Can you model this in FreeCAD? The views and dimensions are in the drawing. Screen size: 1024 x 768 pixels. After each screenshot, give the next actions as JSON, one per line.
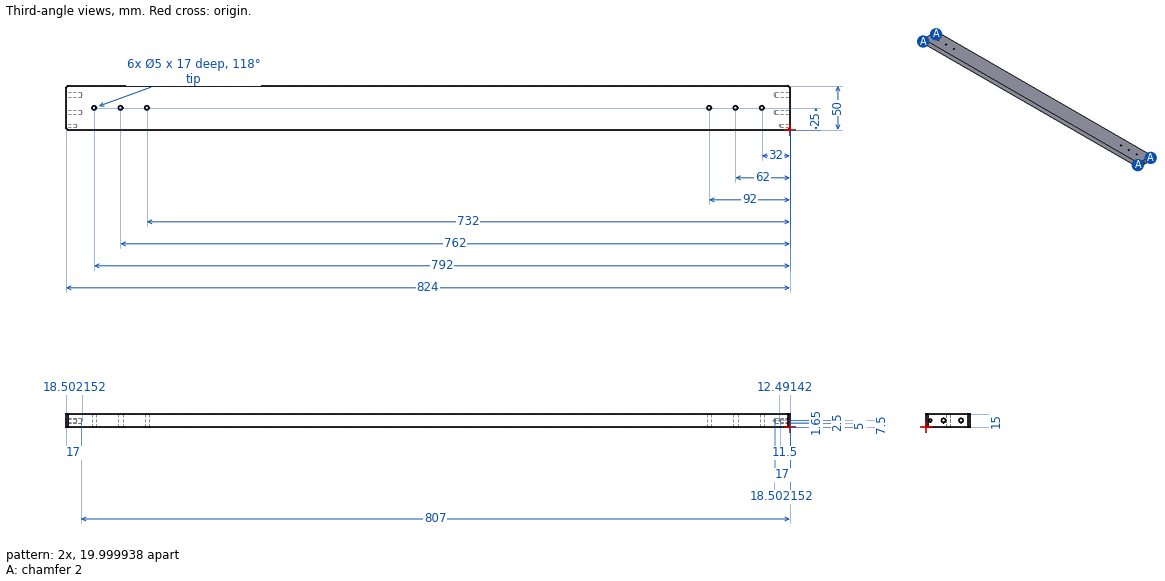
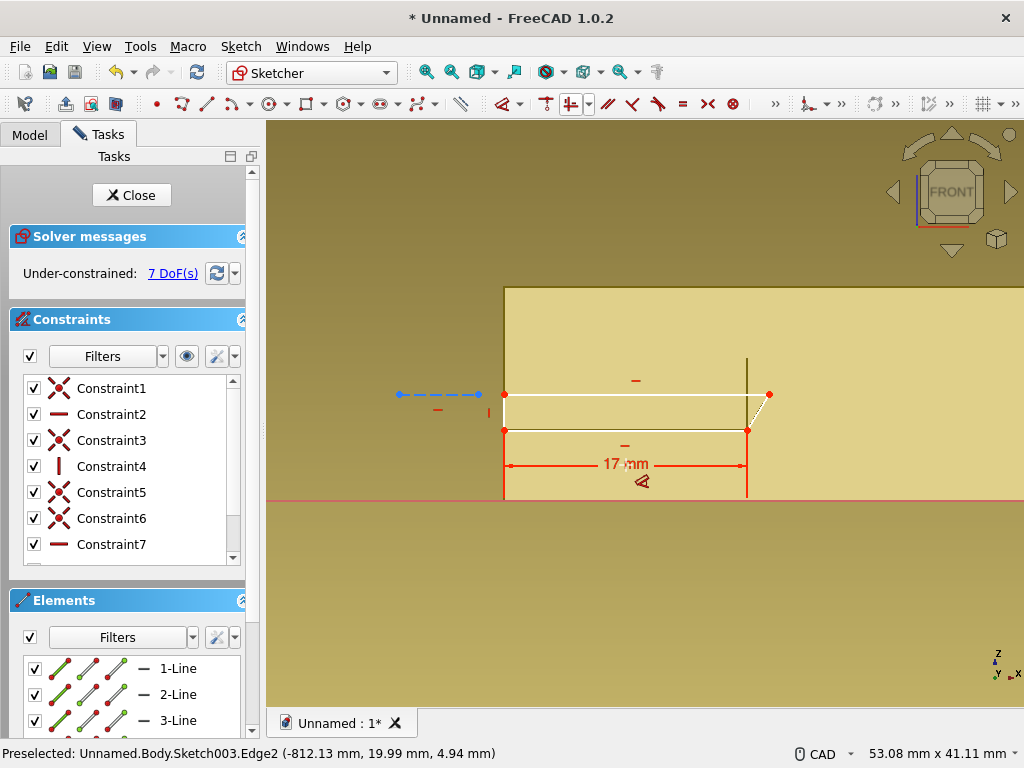
{"action": "left_click", "coordinate": [747, 431]}
{"action": "left_click", "coordinate": [713, 466]}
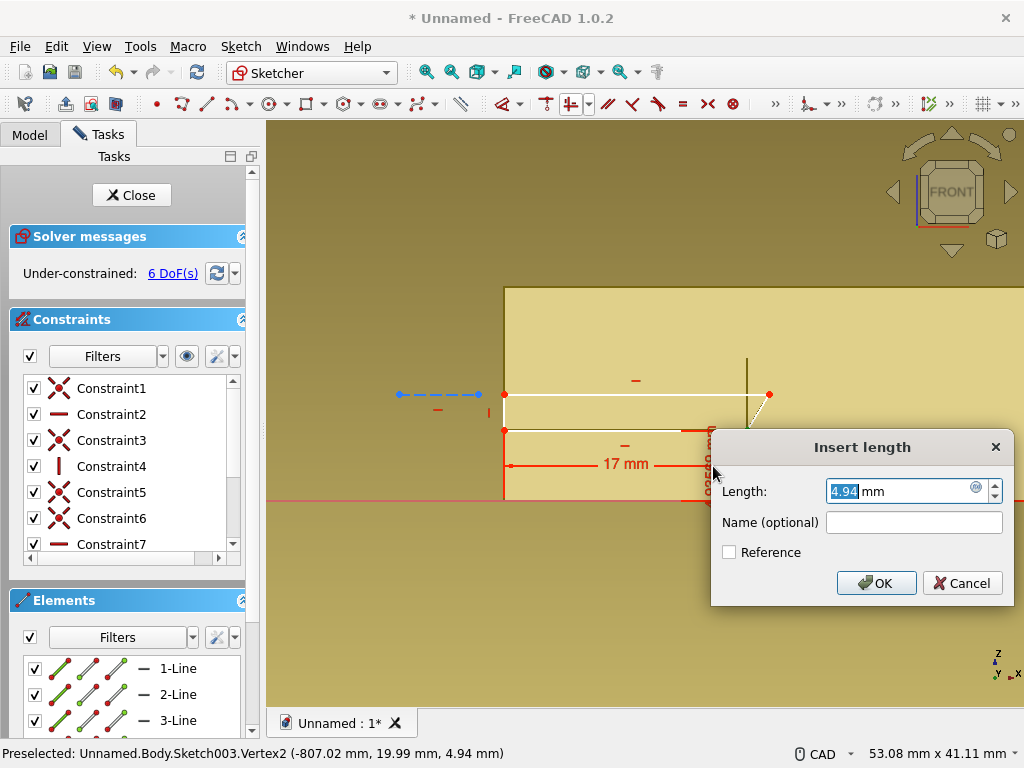
{"action": "type", "text": "5"}
{"action": "key", "text": "Return"}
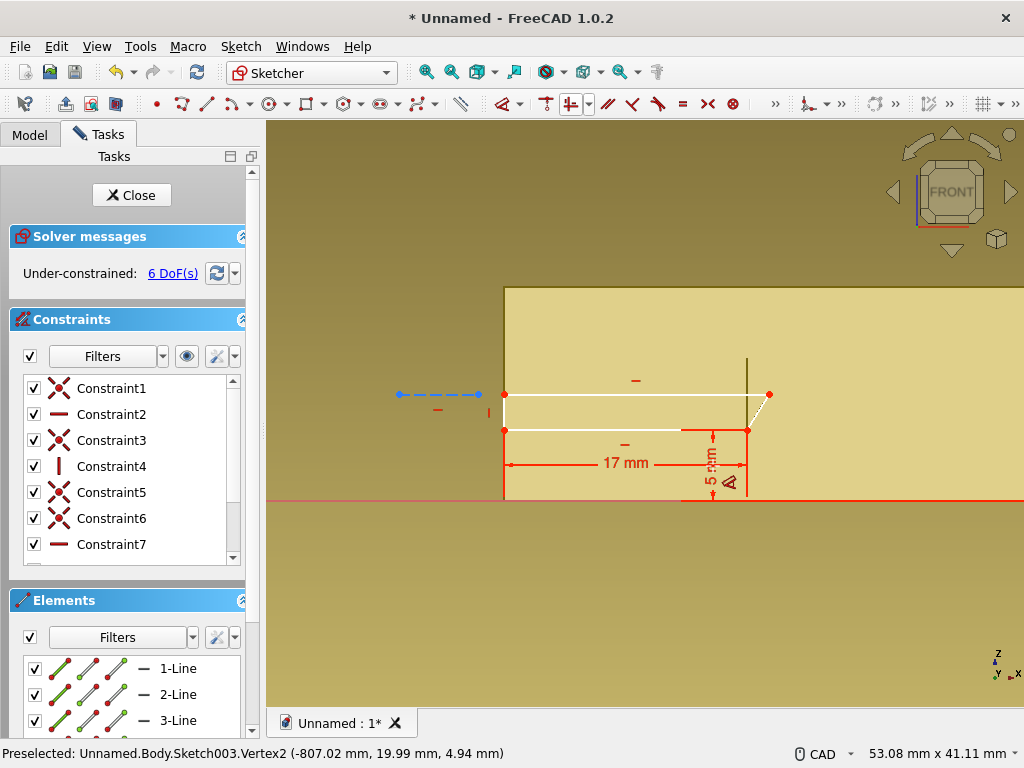
{"action": "scroll", "coordinate": [504, 420], "scroll_direction": "up", "scroll_amount": 2}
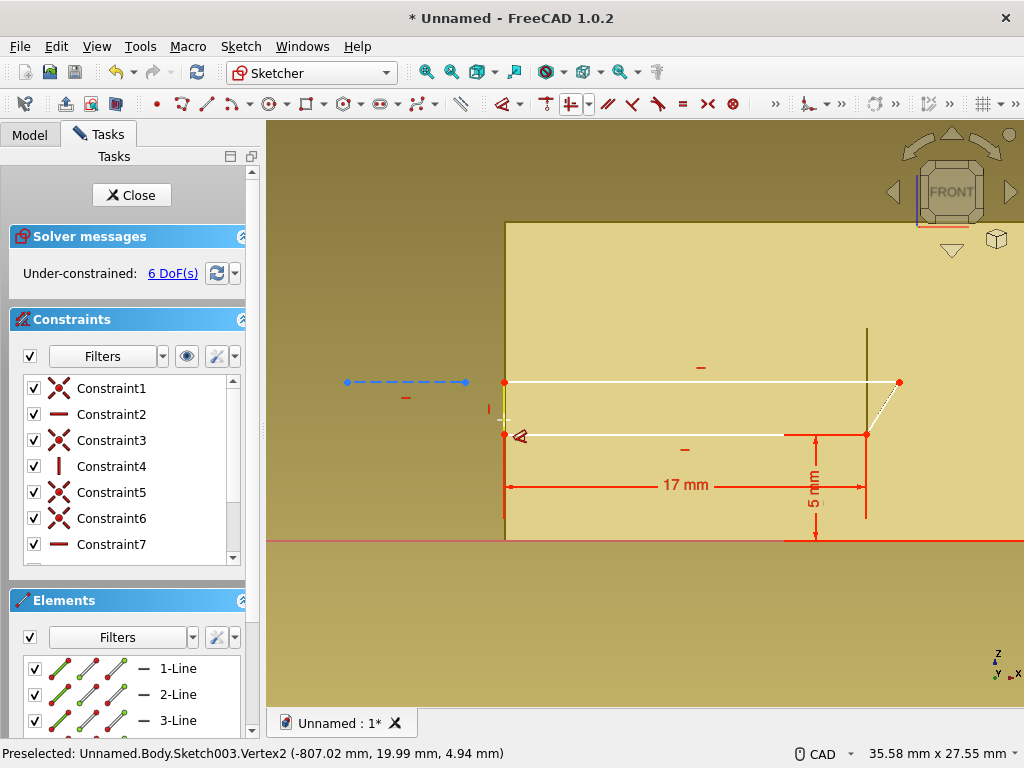
{"action": "left_click", "coordinate": [504, 419]}
{"action": "left_click", "coordinate": [470, 409]}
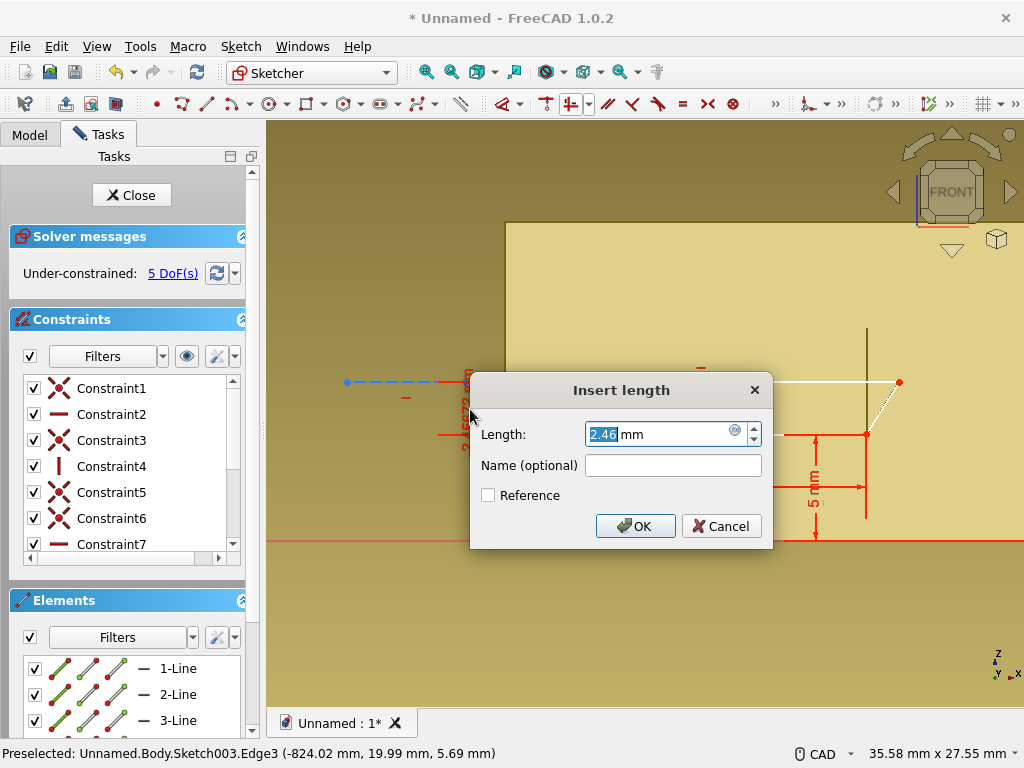
{"action": "type", "text": "2.5"}
{"action": "key", "text": "Return"}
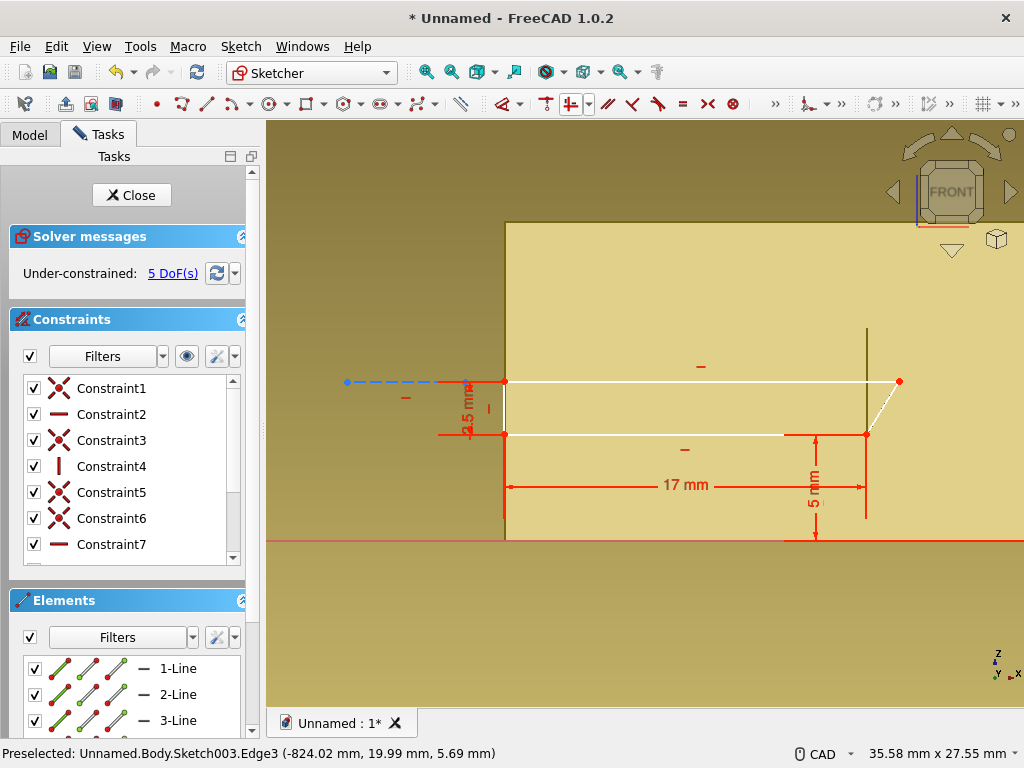
{"action": "scroll", "coordinate": [482, 424], "scroll_direction": "down", "scroll_amount": 2}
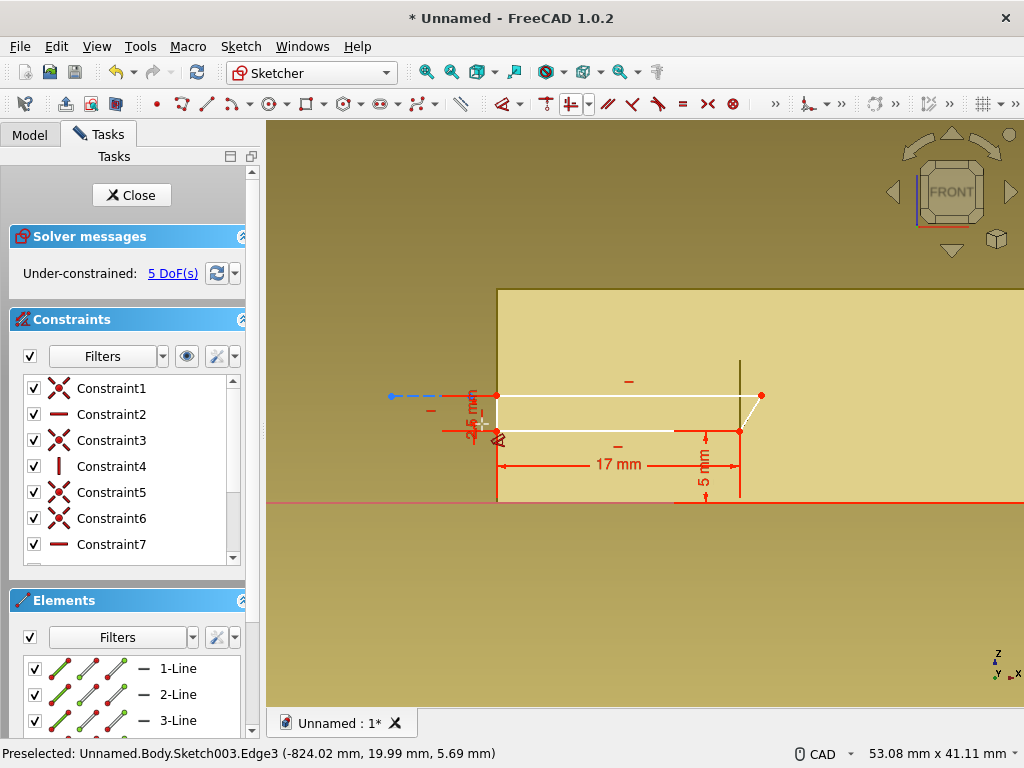
{"action": "left_click", "coordinate": [740, 431]}
{"action": "left_click", "coordinate": [799, 537]}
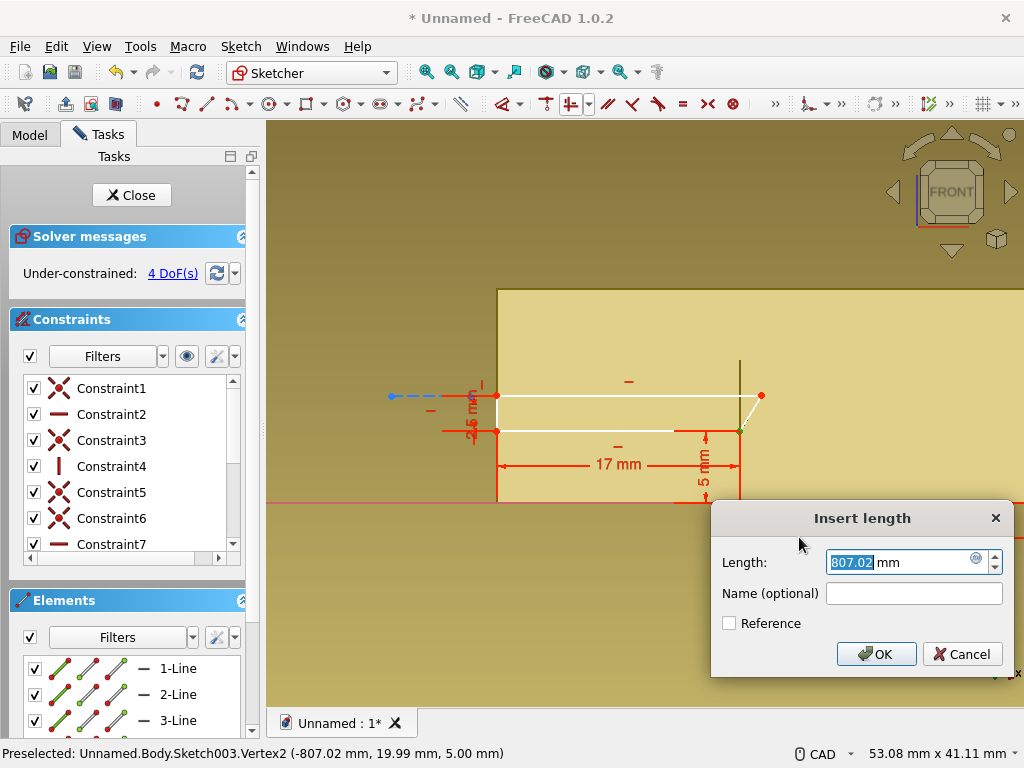
{"action": "type", "text": "807"}
{"action": "key", "text": "Return"}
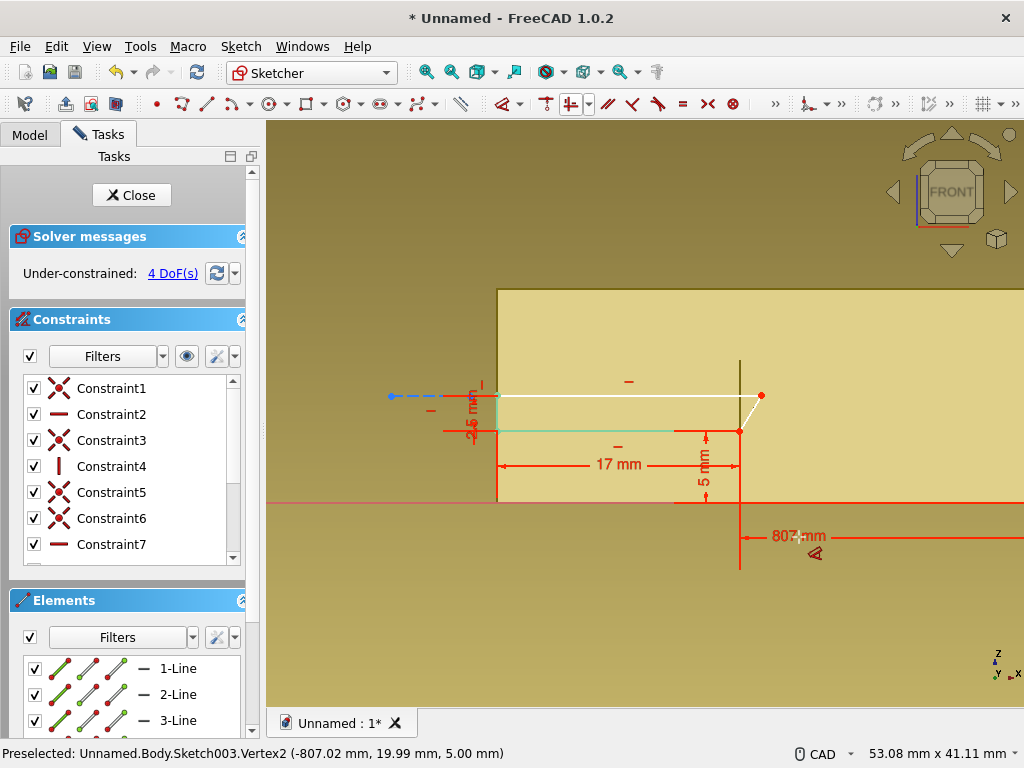
{"action": "left_click", "coordinate": [471, 396]}
{"action": "left_click", "coordinate": [437, 450]}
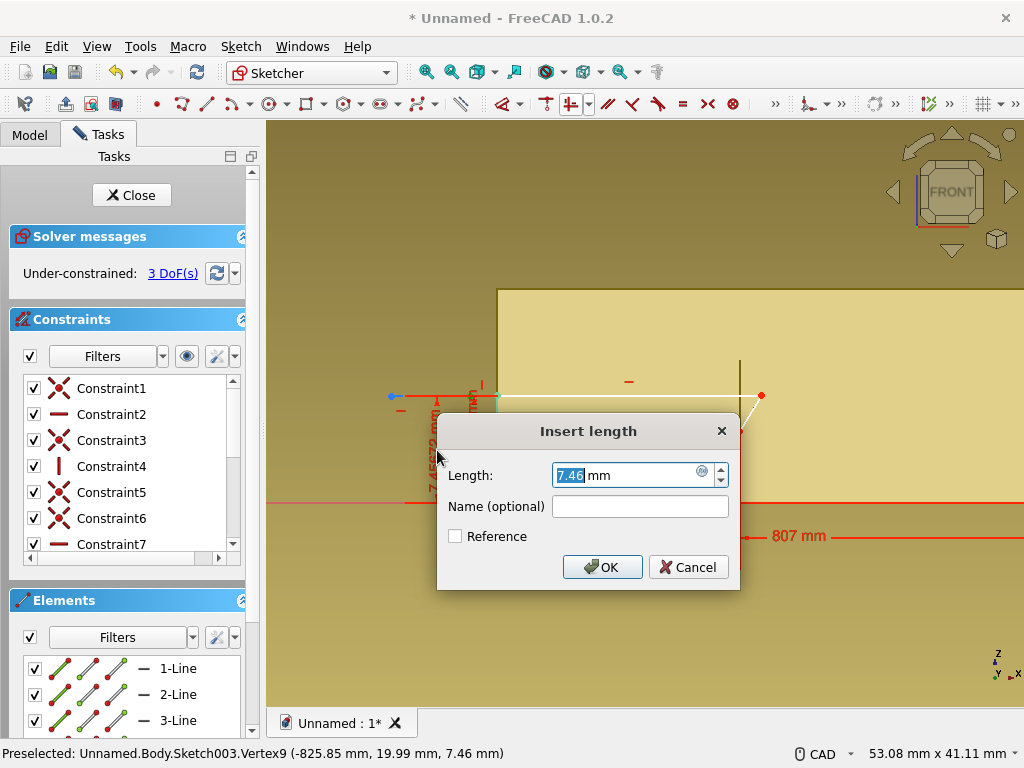
{"action": "type", "text": "7.5"}
{"action": "key", "text": "Return"}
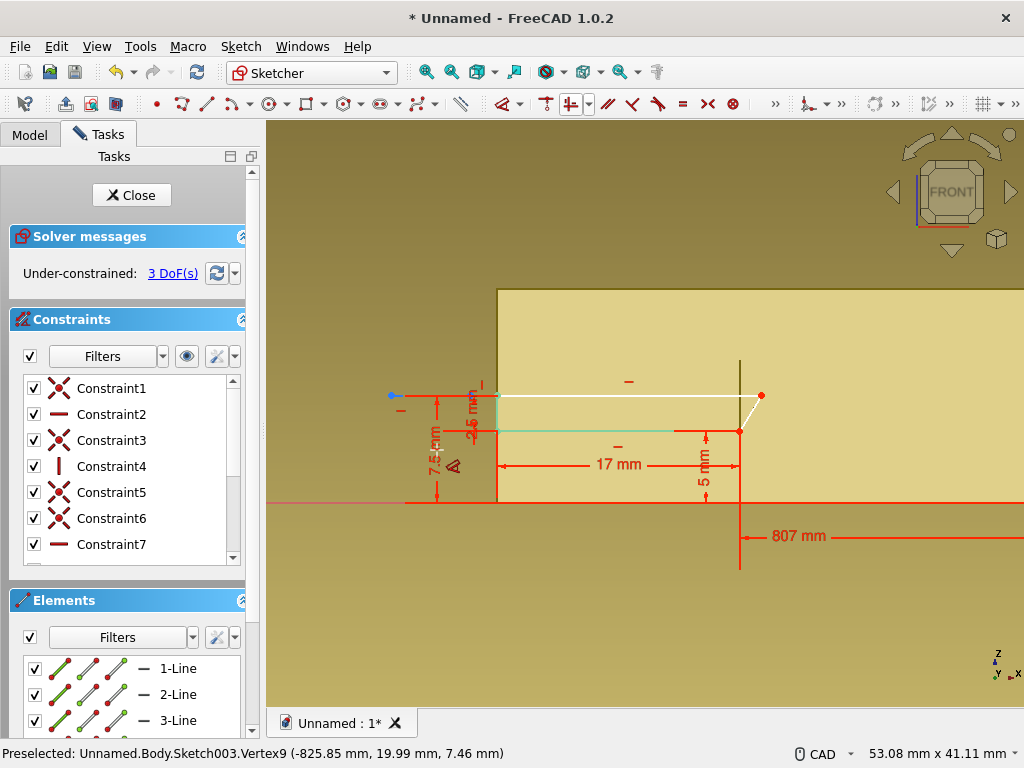
{"action": "left_click", "coordinate": [577, 396]}
{"action": "left_click", "coordinate": [629, 362]}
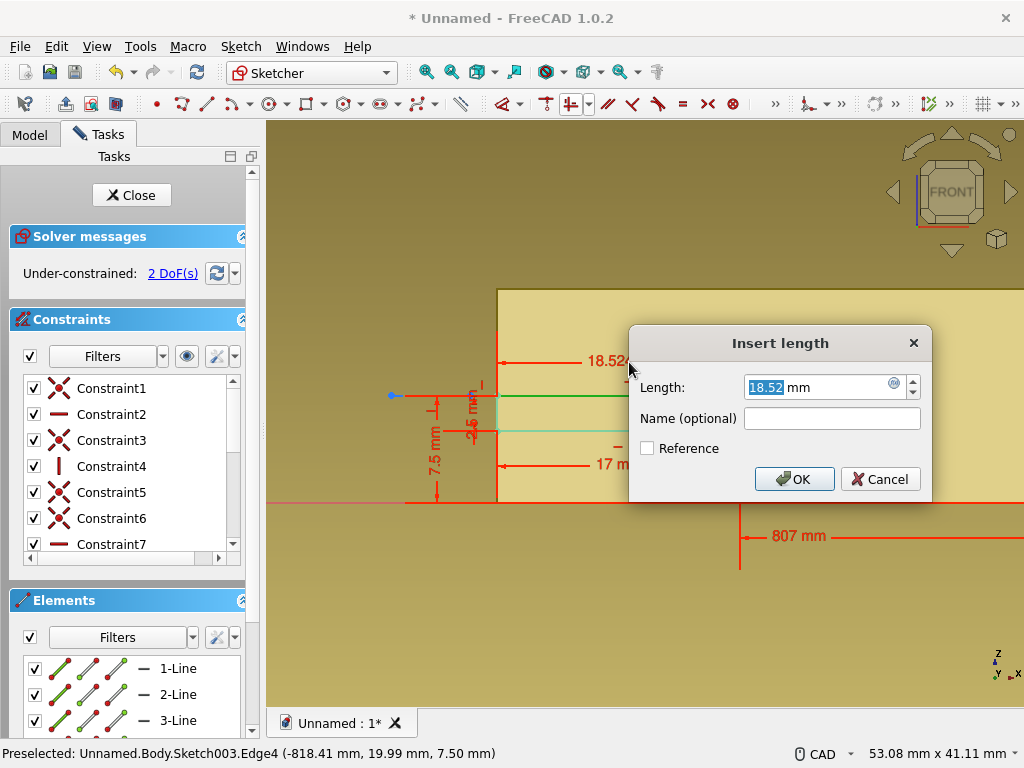
{"action": "type", "text": "18.502152"}
{"action": "key", "text": "Return"}
{"action": "key", "text": "Escape"}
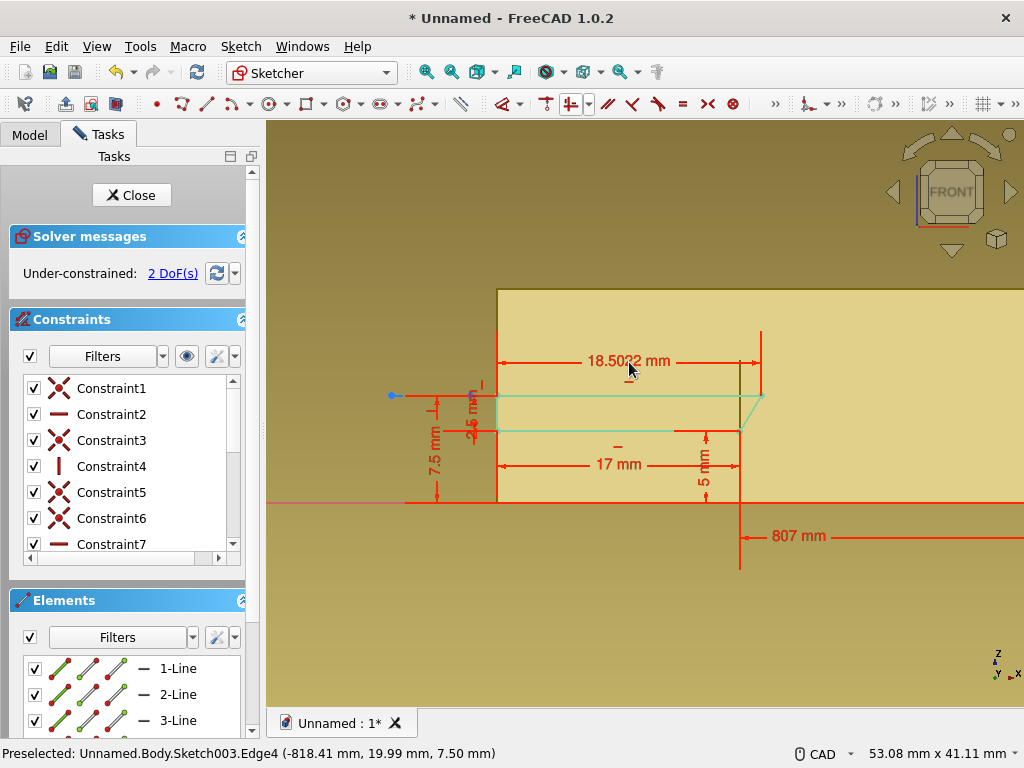
{"action": "left_click", "coordinate": [132, 195]}